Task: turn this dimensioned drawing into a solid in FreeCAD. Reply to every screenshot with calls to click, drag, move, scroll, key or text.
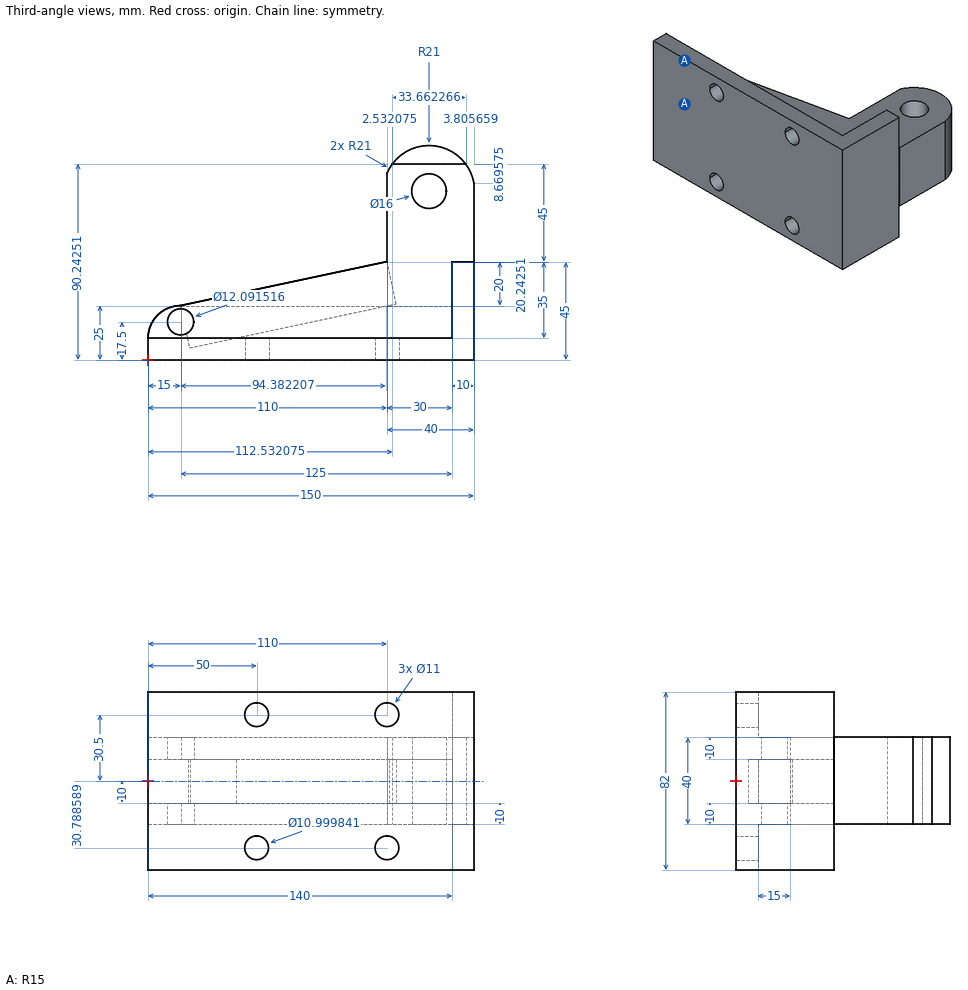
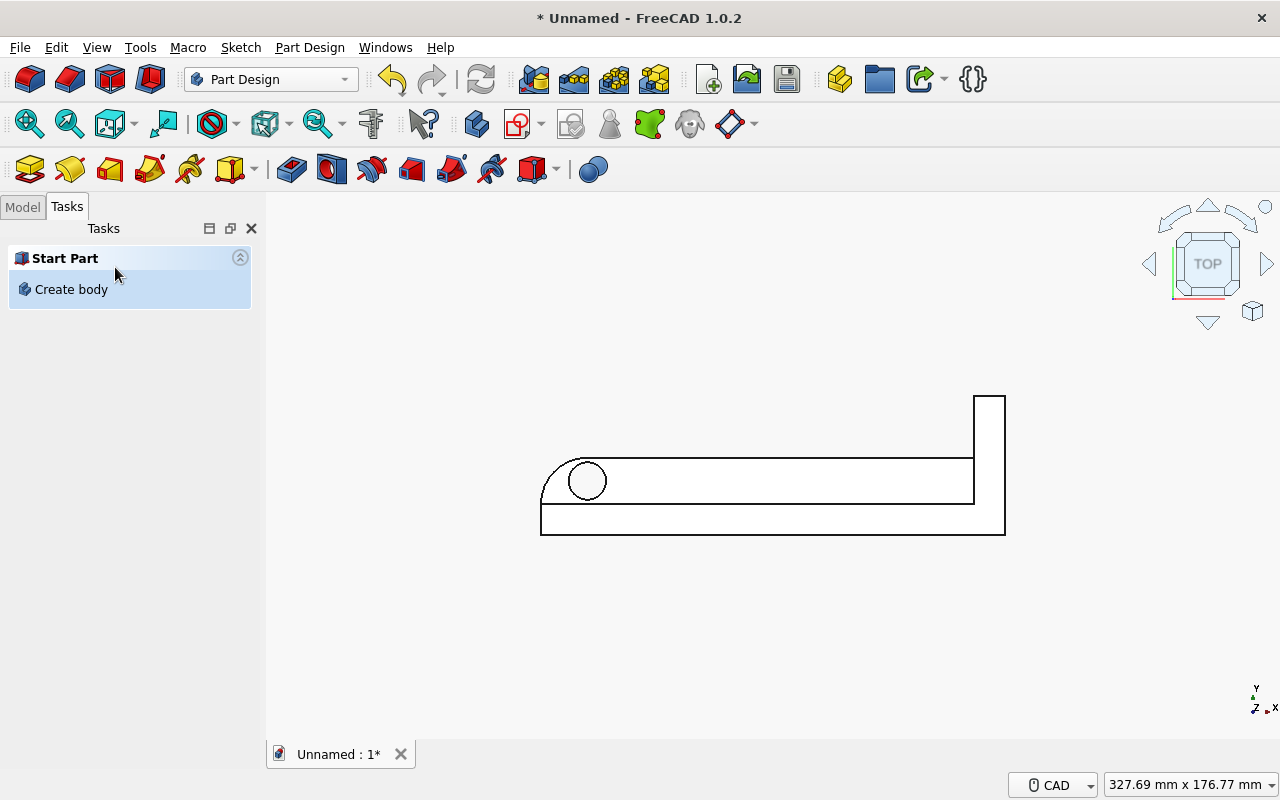
click(943, 480)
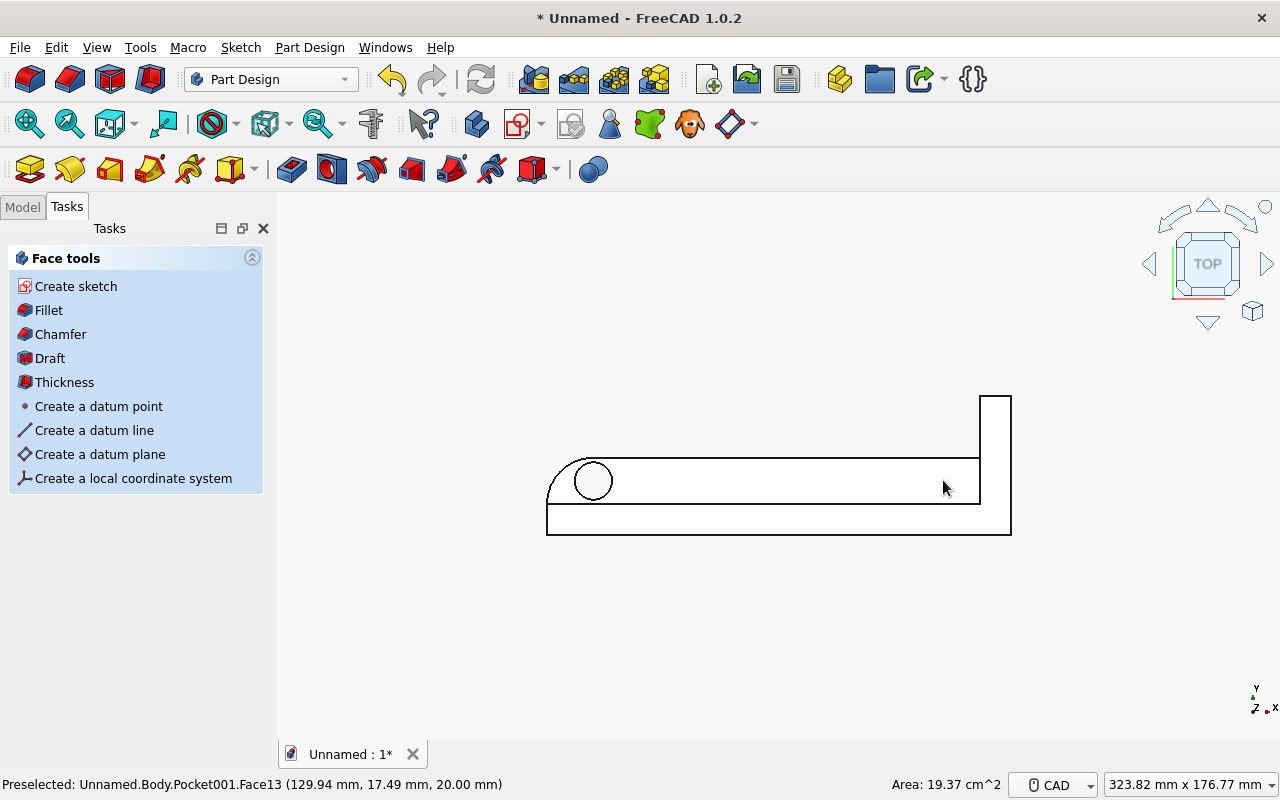
click(518, 124)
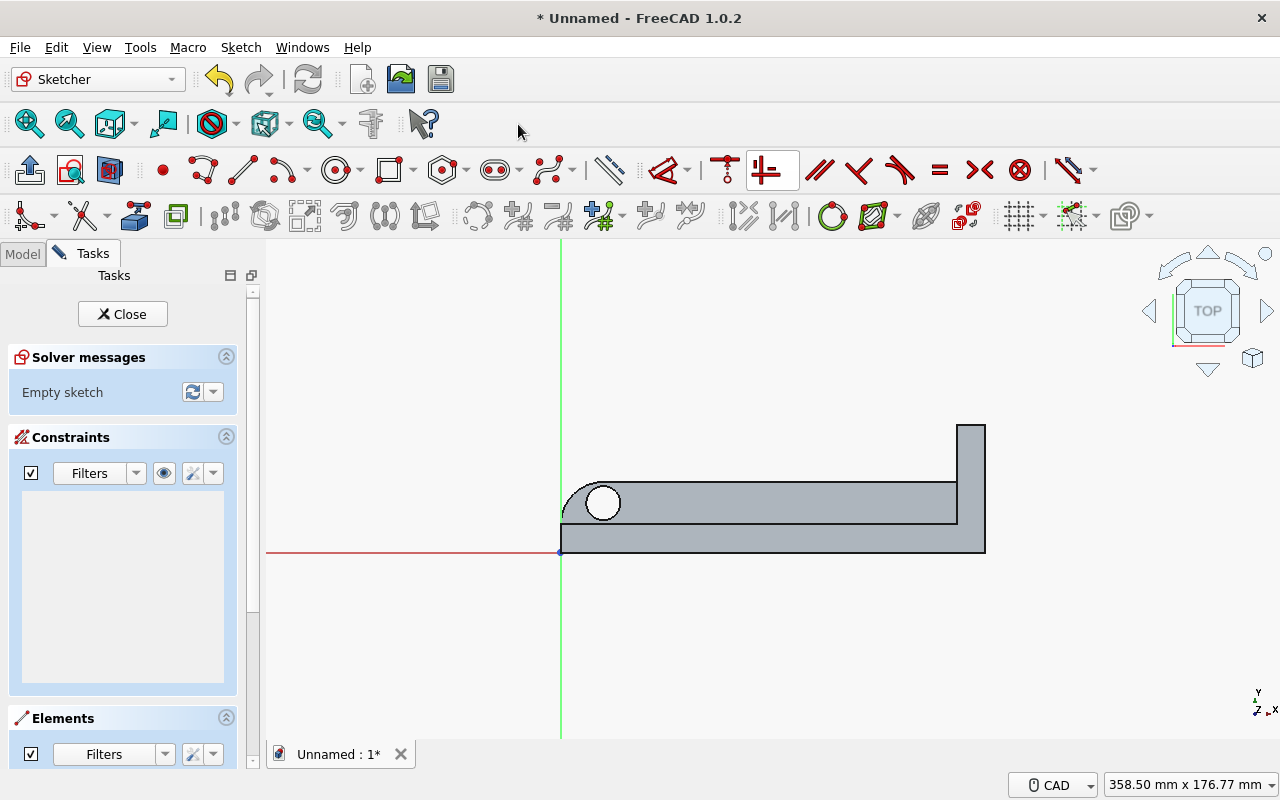
scroll(729, 489, up, 3)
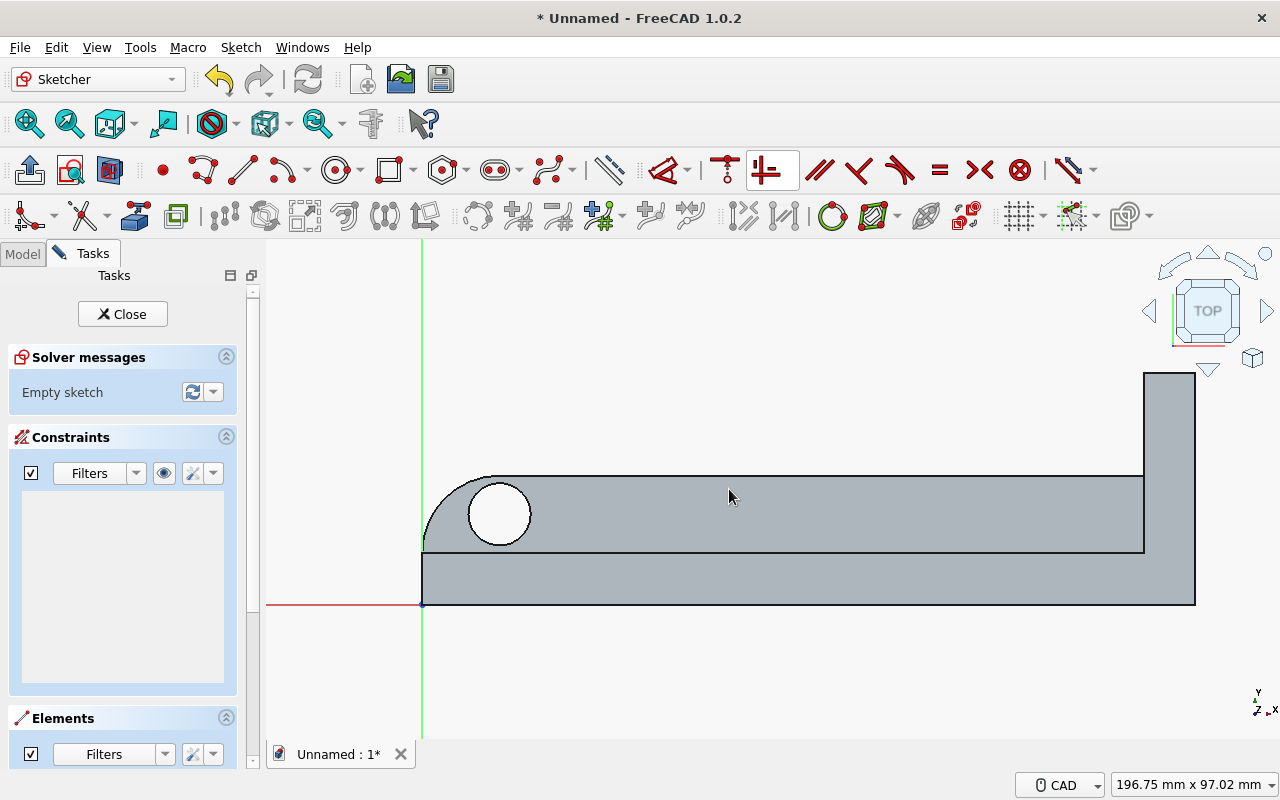
key(g)
key(m)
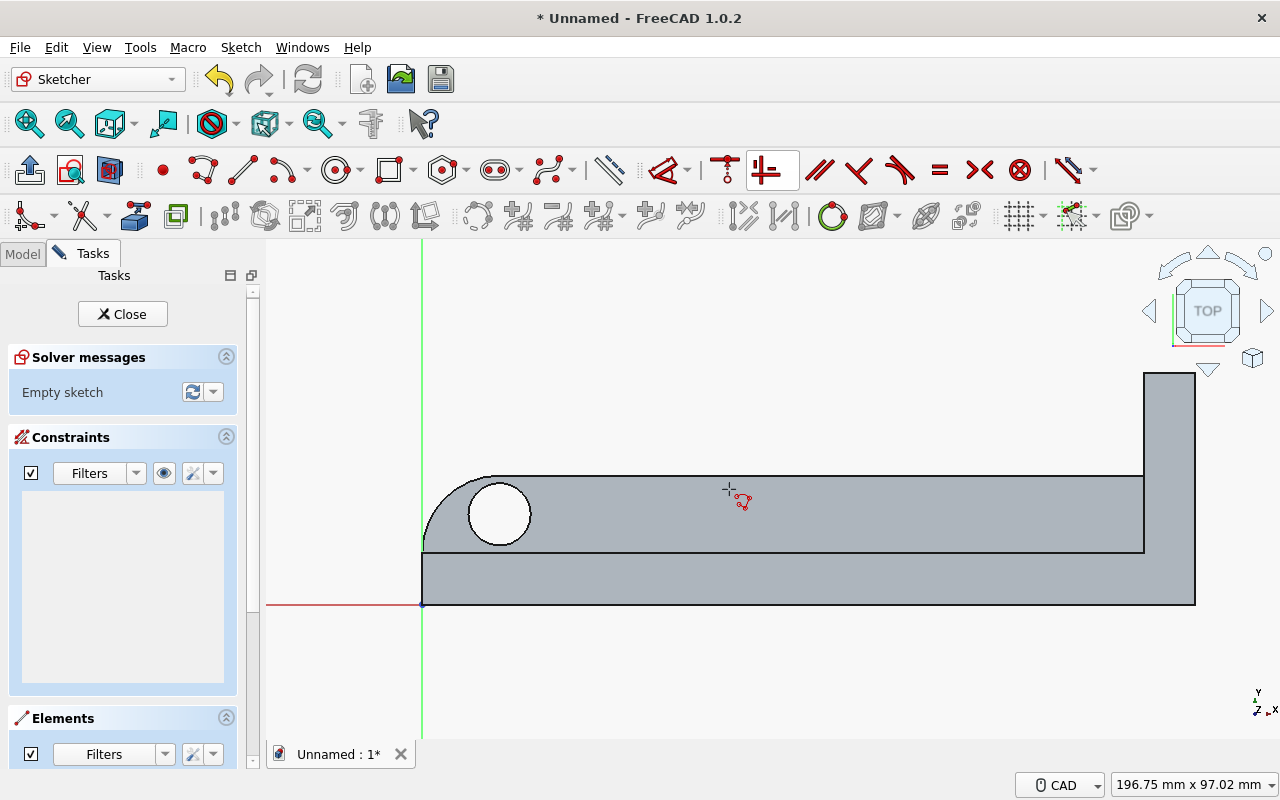
click(500, 476)
click(986, 476)
click(986, 373)
click(500, 477)
key(Escape)
key(Escape)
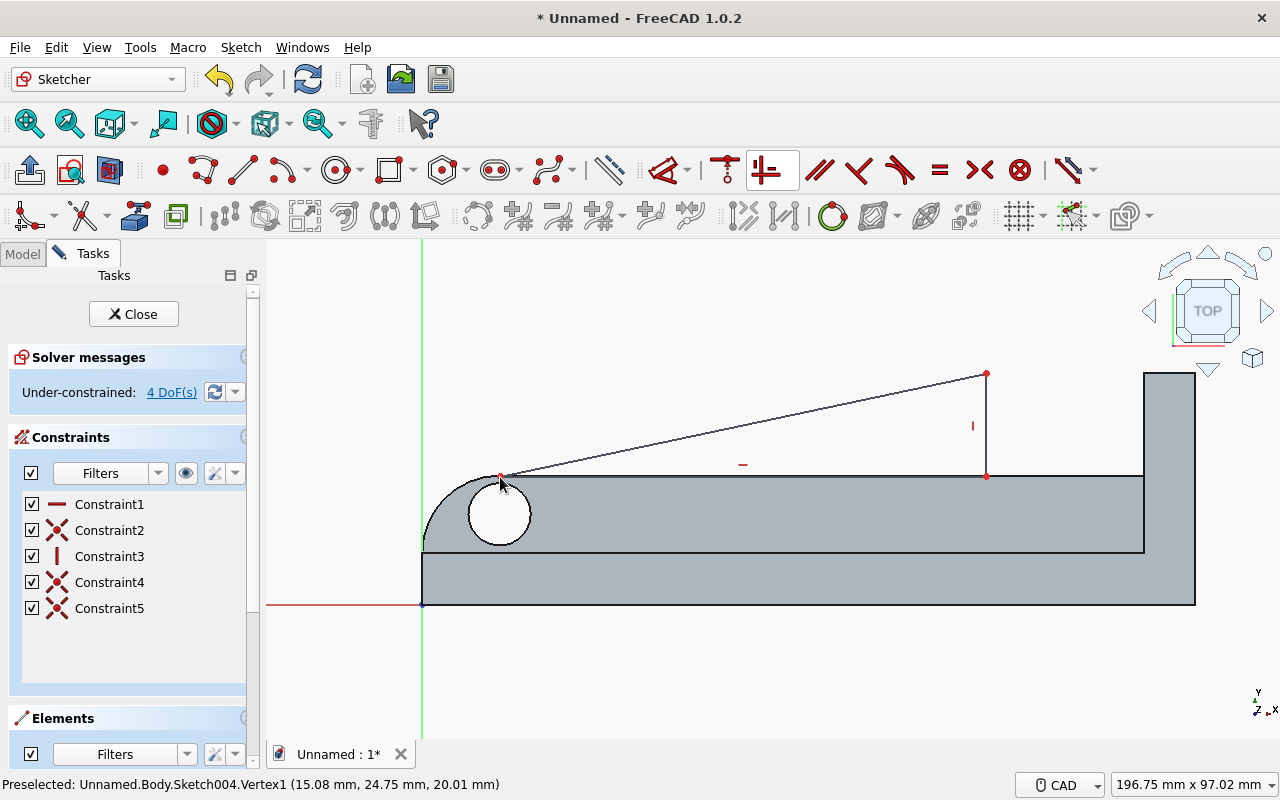
key(d)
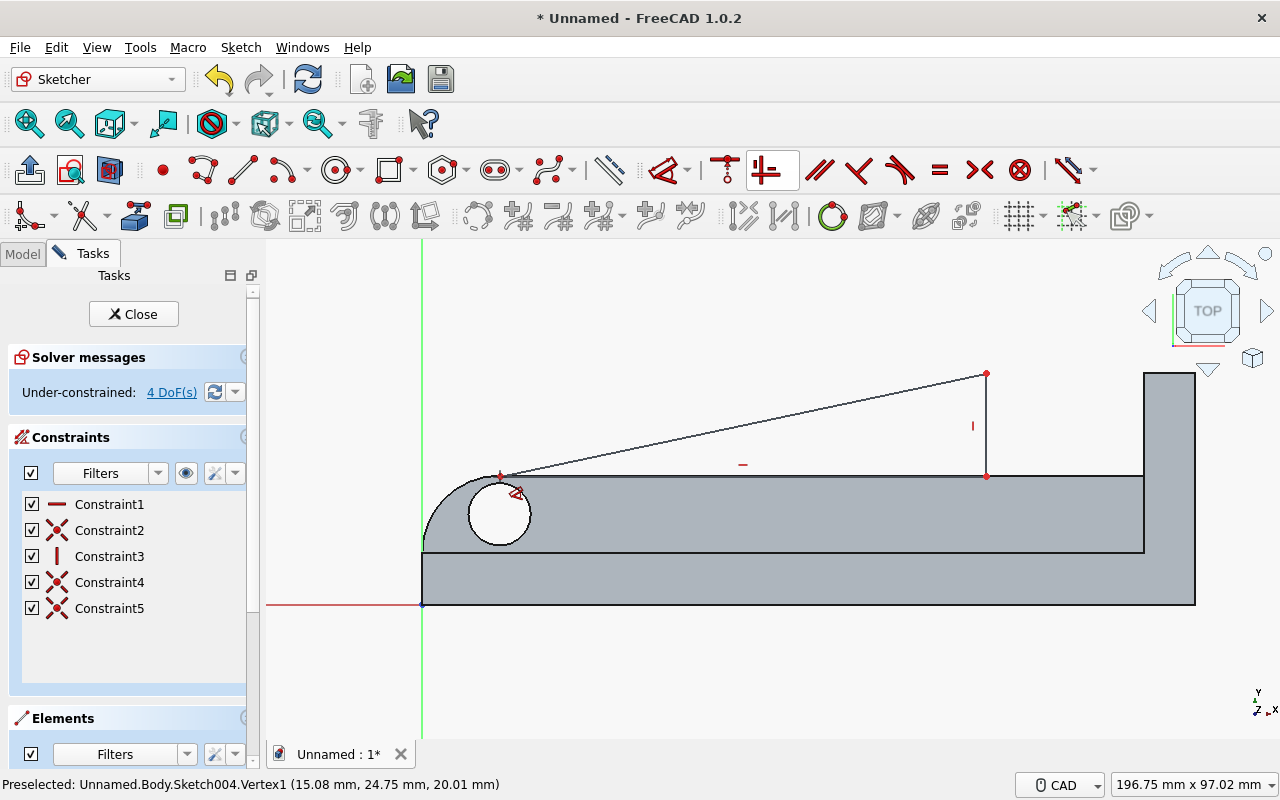
click(986, 446)
click(1020, 425)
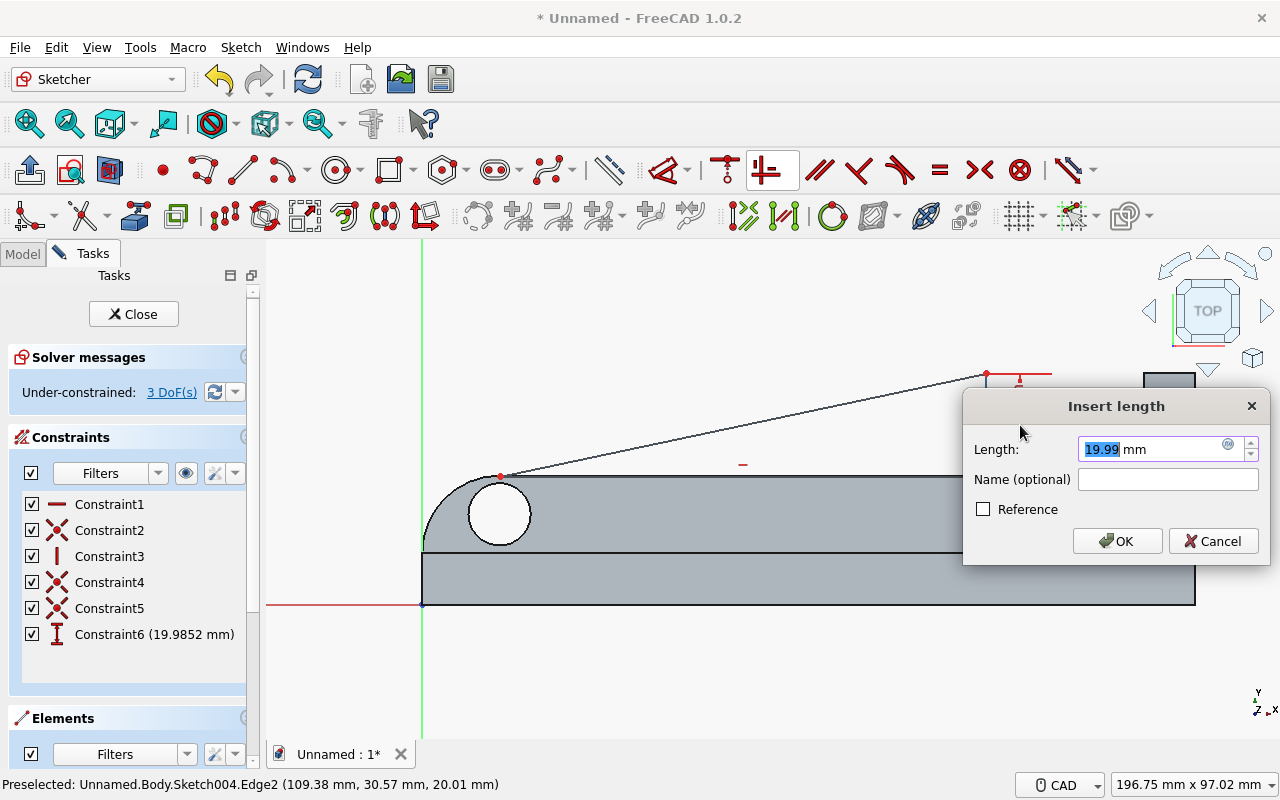
text(20)
key(Return)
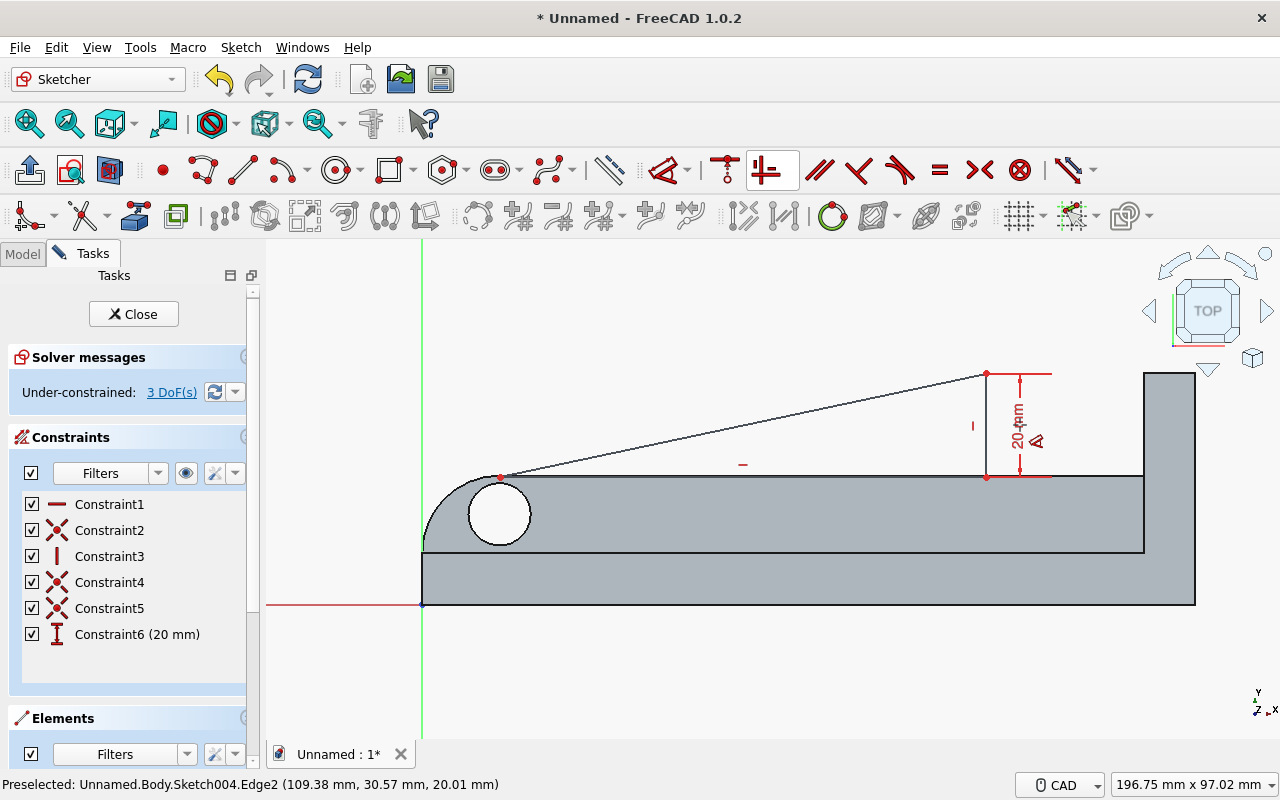
click(500, 477)
click(461, 639)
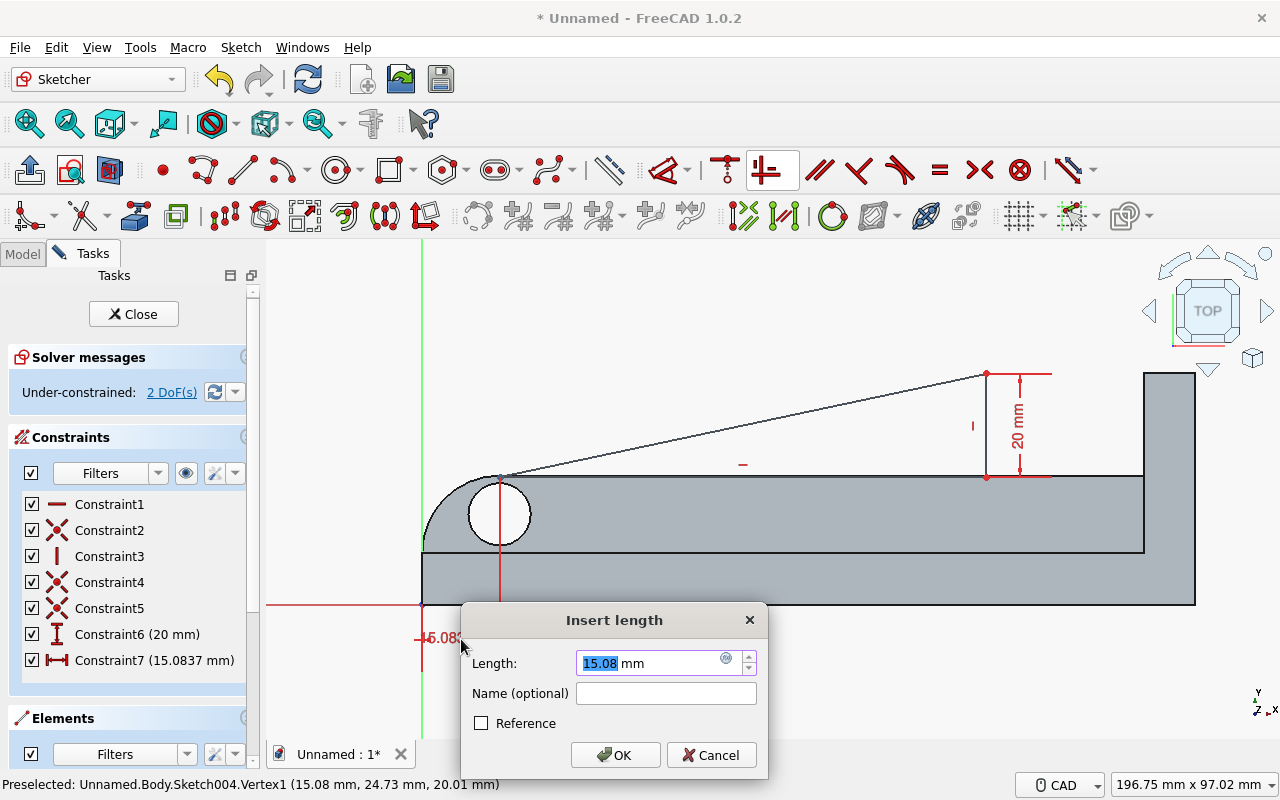
text(15)
key(Return)